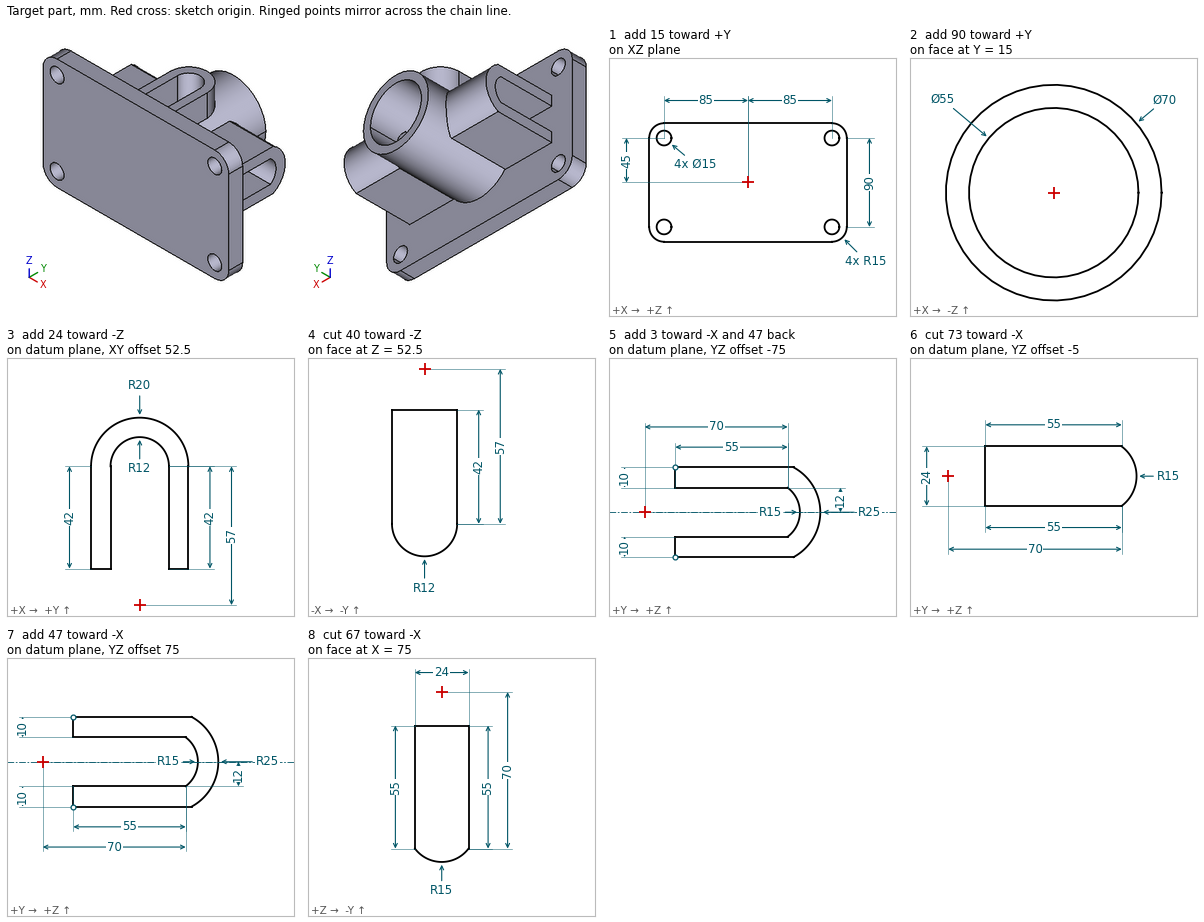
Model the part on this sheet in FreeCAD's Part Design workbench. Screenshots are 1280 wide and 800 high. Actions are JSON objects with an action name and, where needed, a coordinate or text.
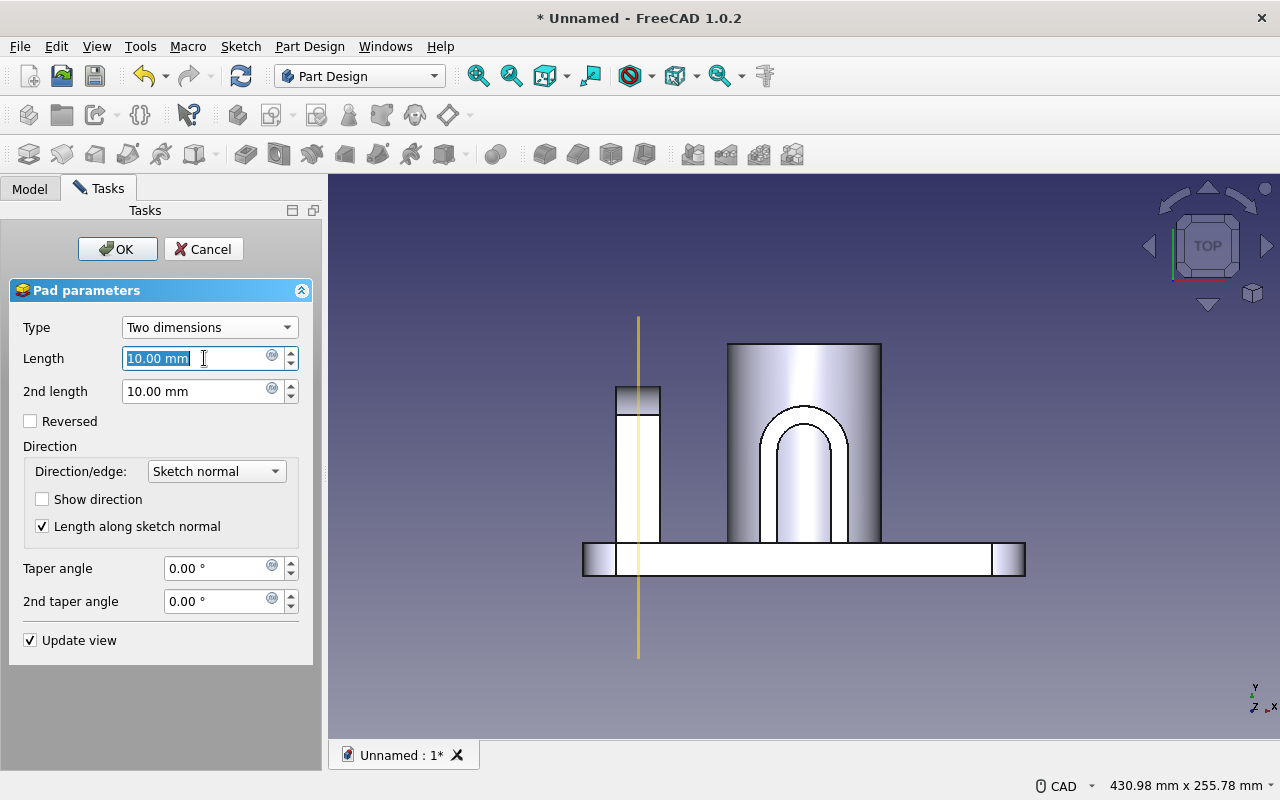
{"action": "type", "text": "3"}
{"action": "key", "text": "Tab"}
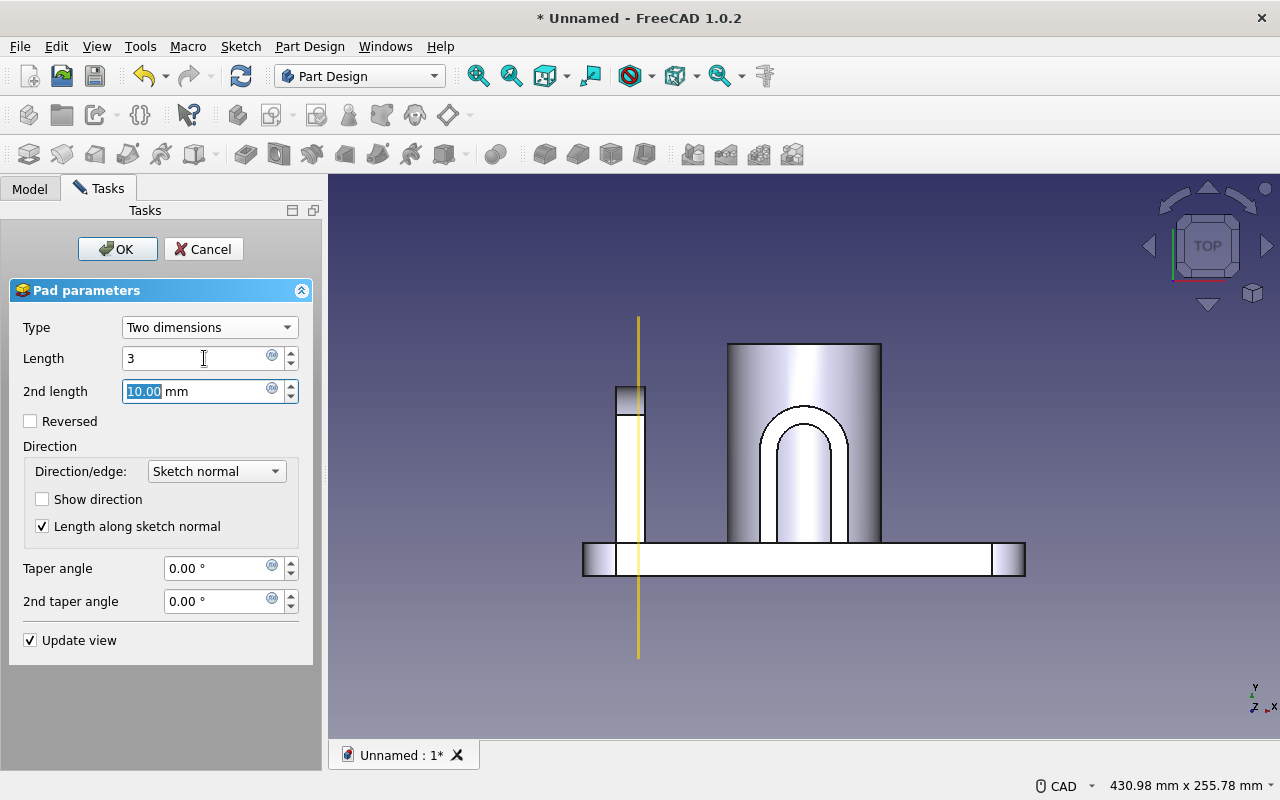
{"action": "type", "text": "47"}
{"action": "key", "text": "Tab"}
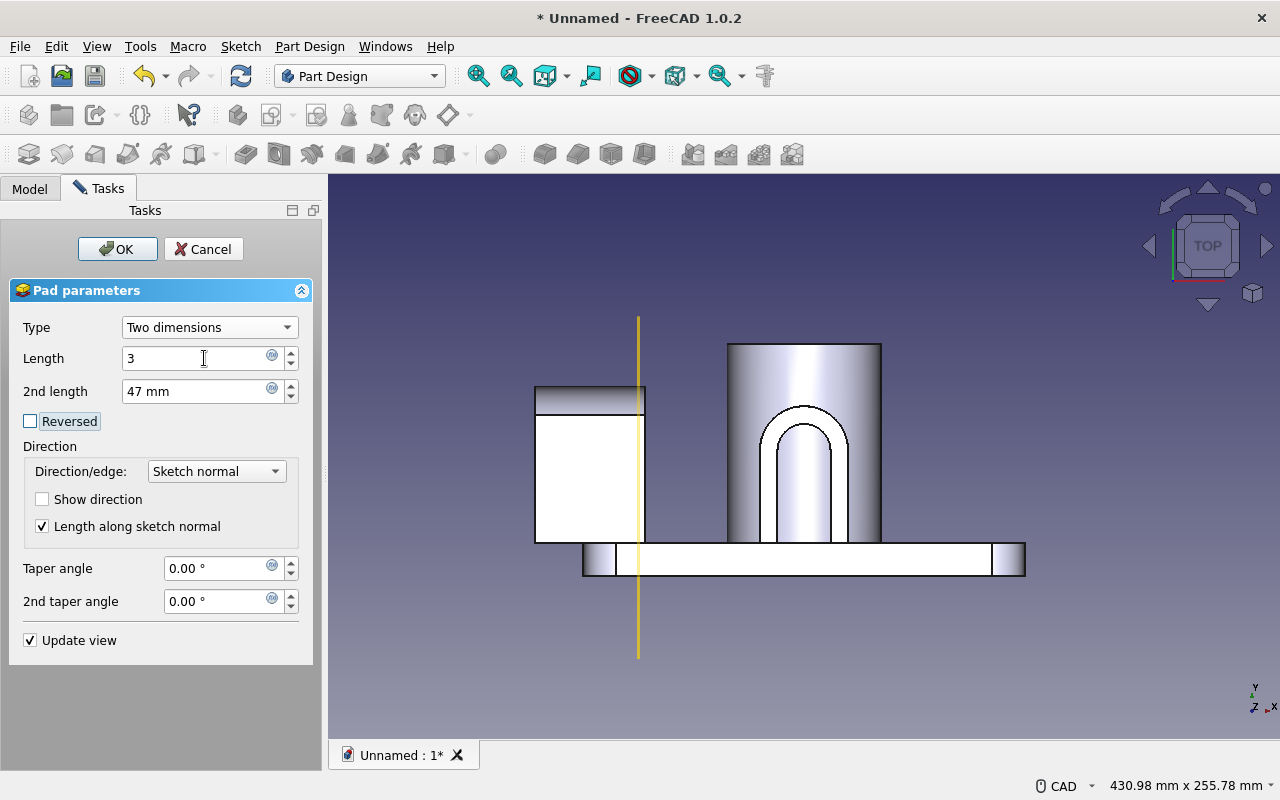
{"action": "left_click", "coordinate": [31, 421]}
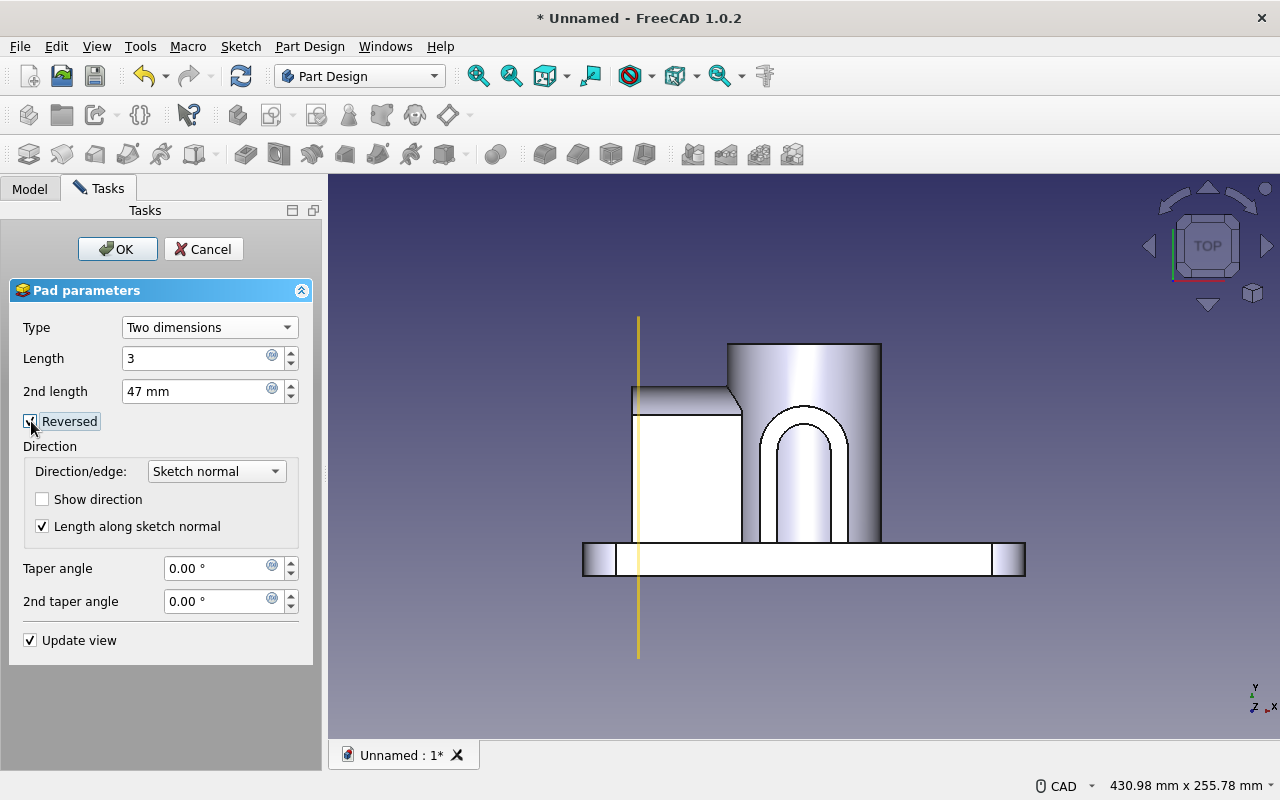
{"action": "left_click", "coordinate": [118, 249]}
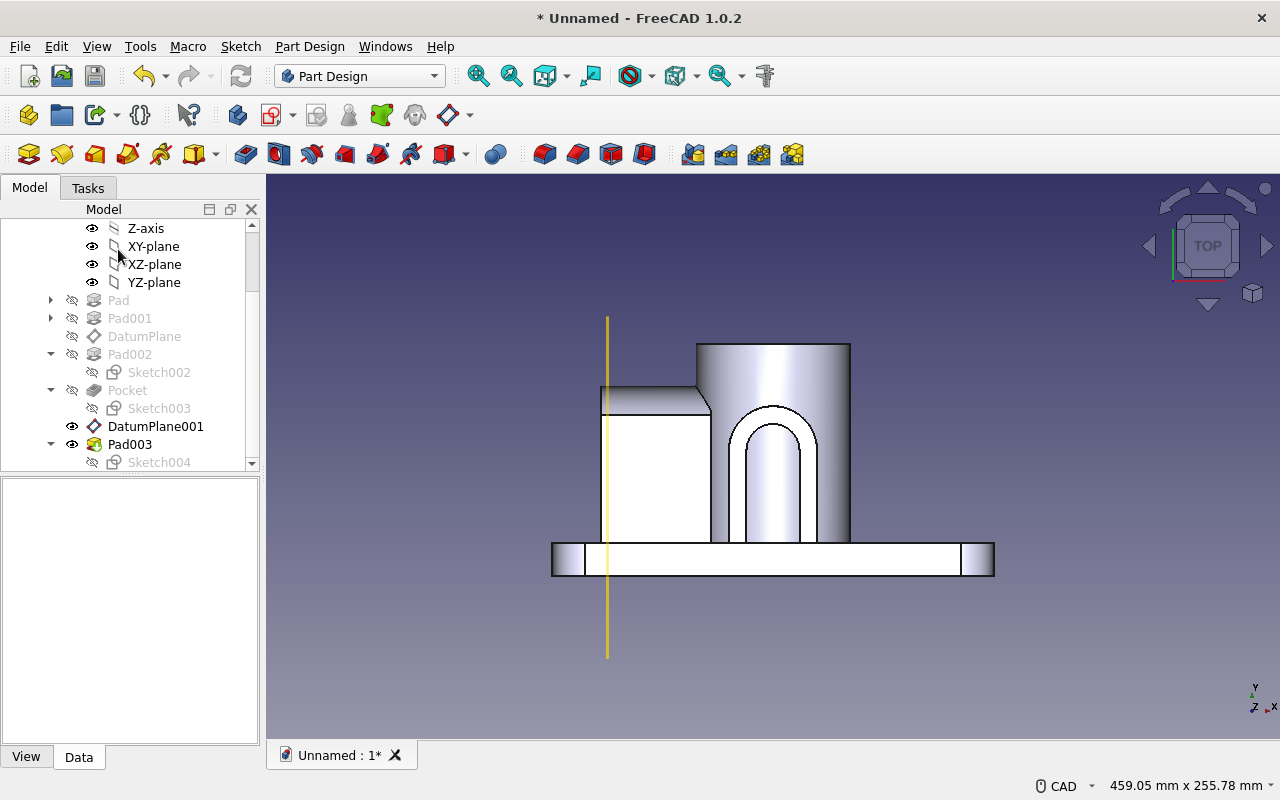
{"action": "left_click", "coordinate": [117, 426]}
{"action": "key", "text": "space"}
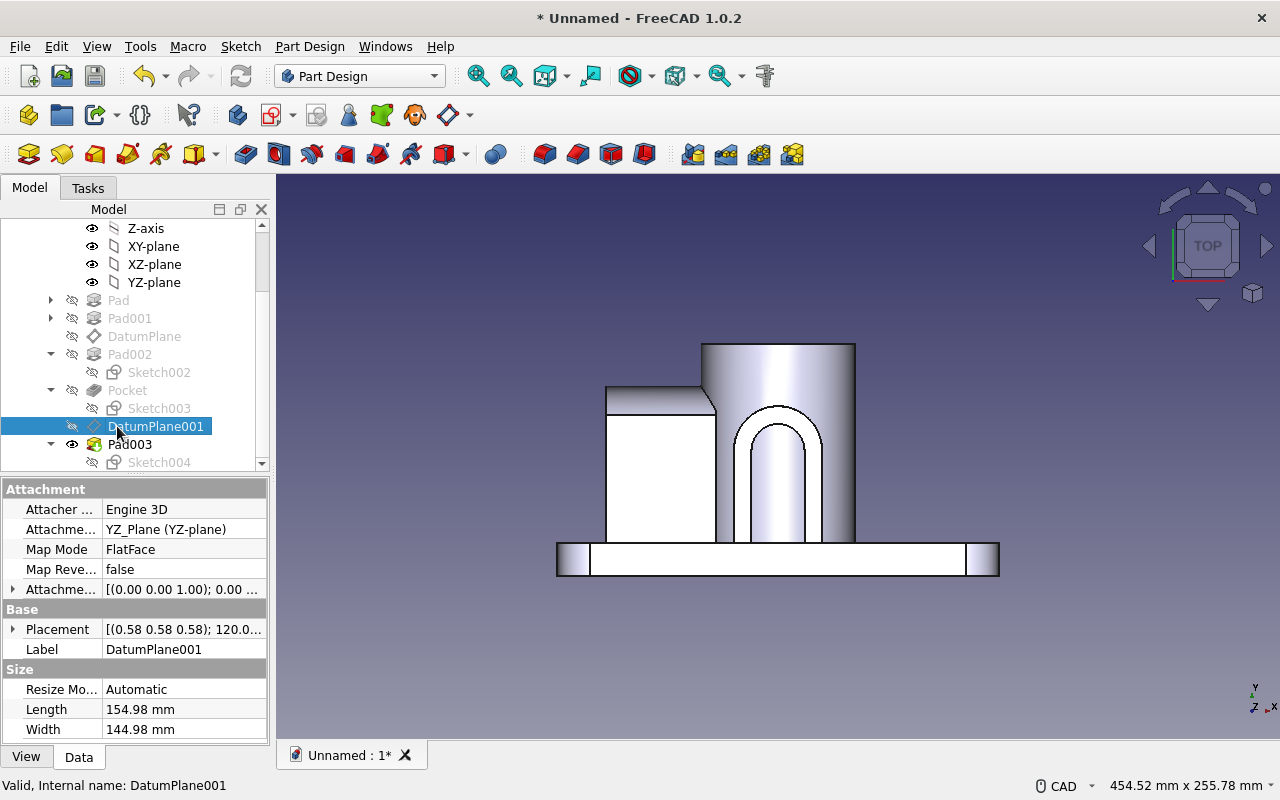
{"action": "key", "text": "v f"}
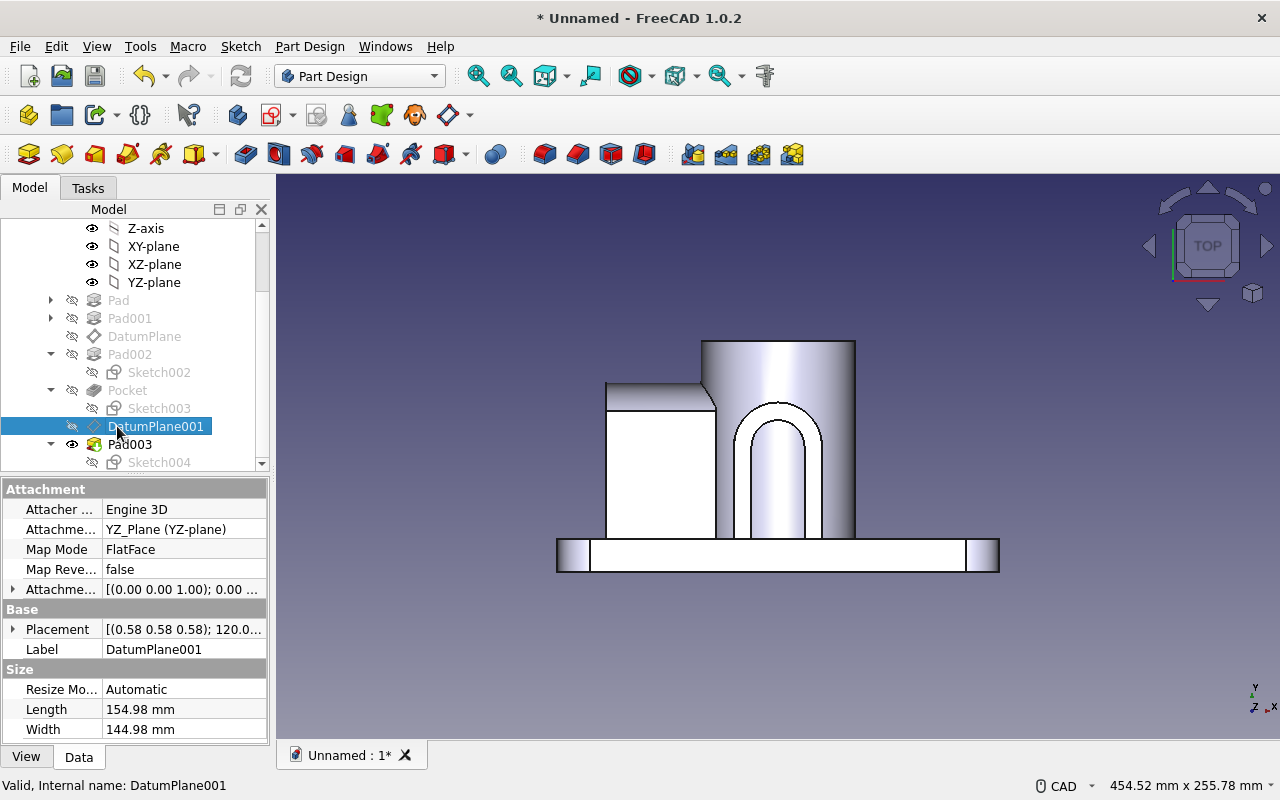
{"action": "scroll", "coordinate": [161, 350], "scroll_direction": "down", "scroll_amount": 3}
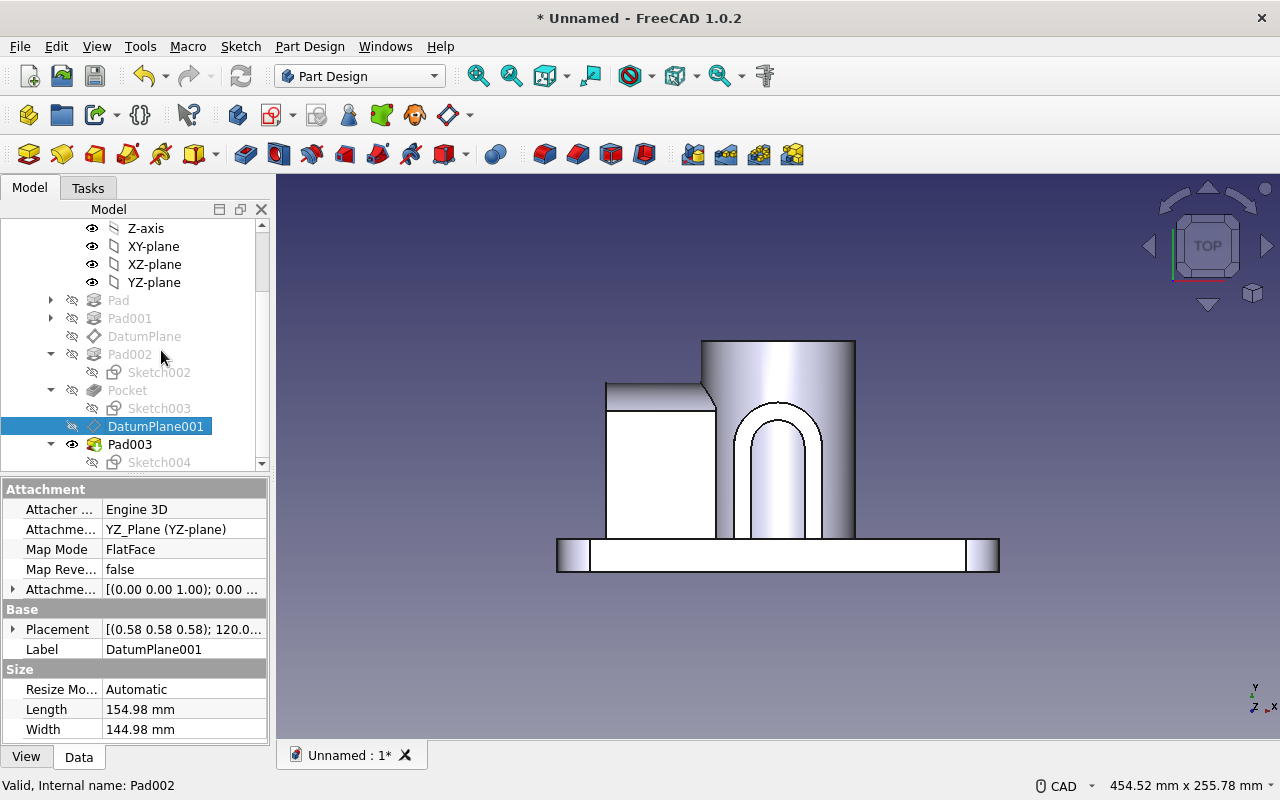
{"action": "scroll", "coordinate": [161, 350], "scroll_direction": "up", "scroll_amount": 15}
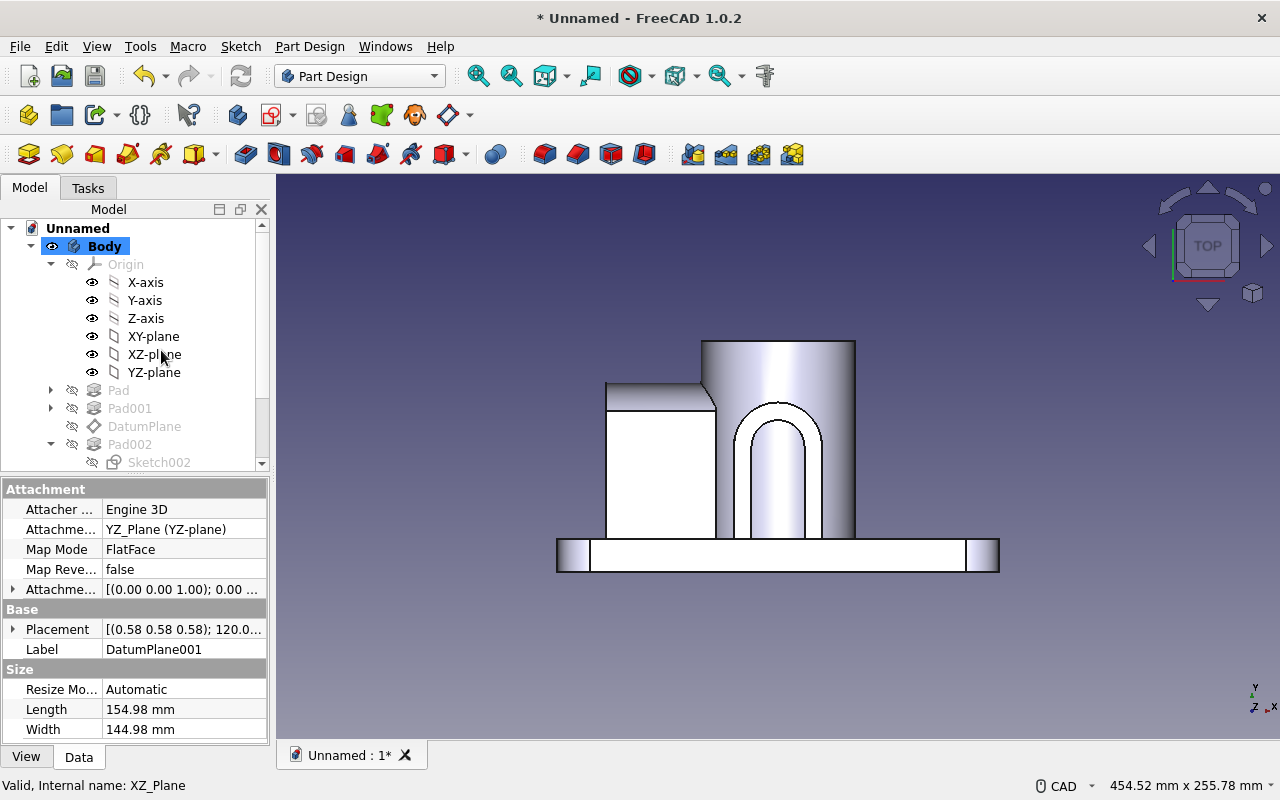
{"action": "left_click", "coordinate": [137, 372]}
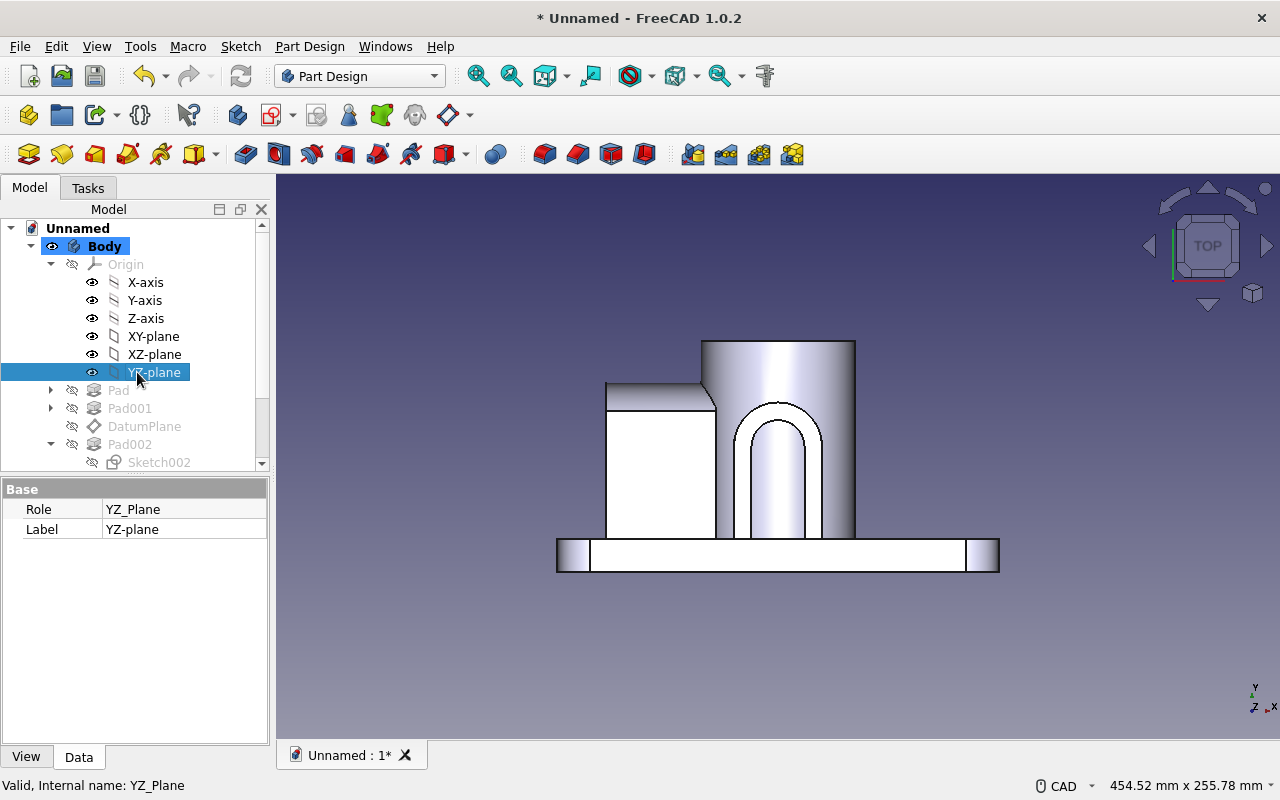
{"action": "left_click", "coordinate": [448, 116]}